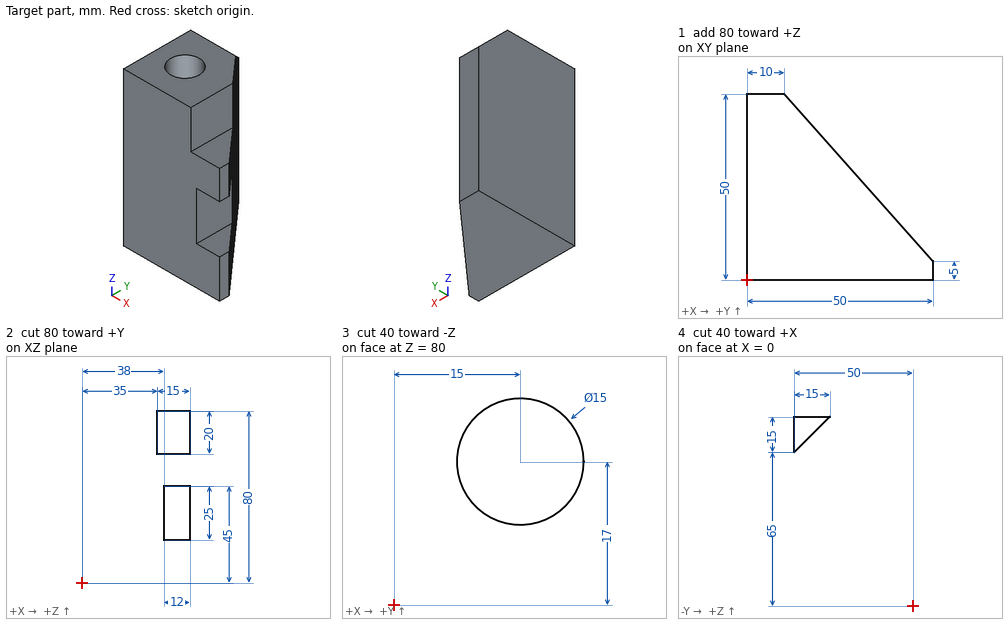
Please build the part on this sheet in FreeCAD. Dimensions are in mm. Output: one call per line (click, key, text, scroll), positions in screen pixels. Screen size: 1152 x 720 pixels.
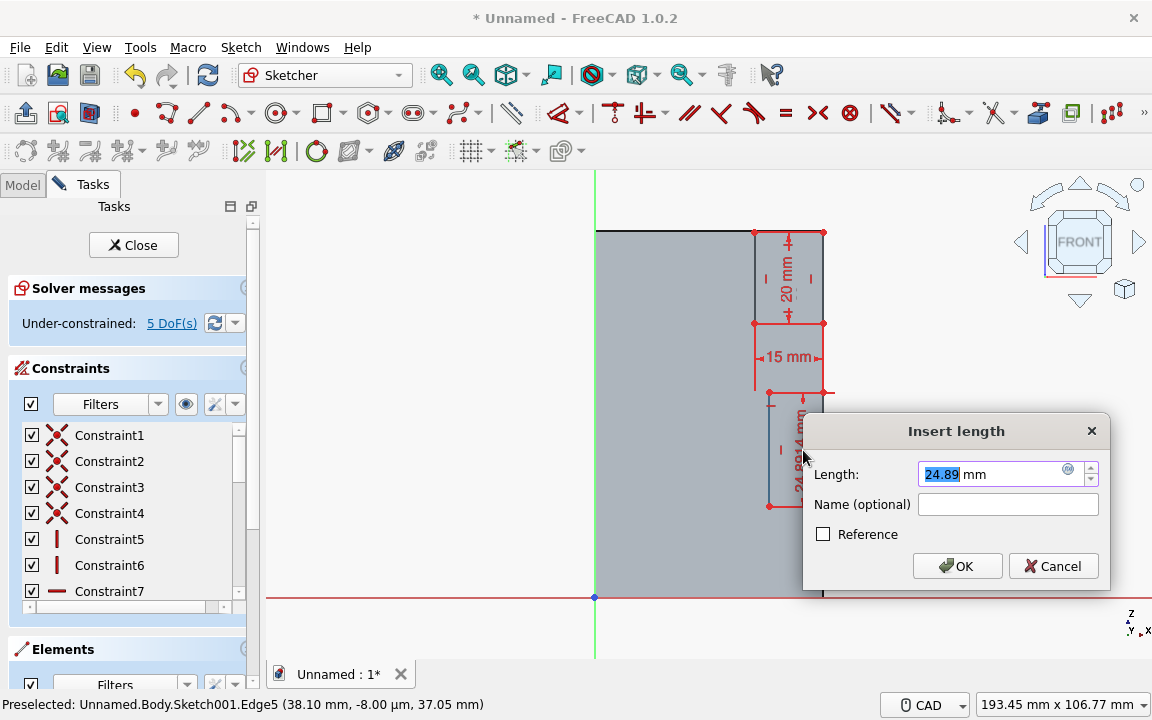
text(25)
key(Return)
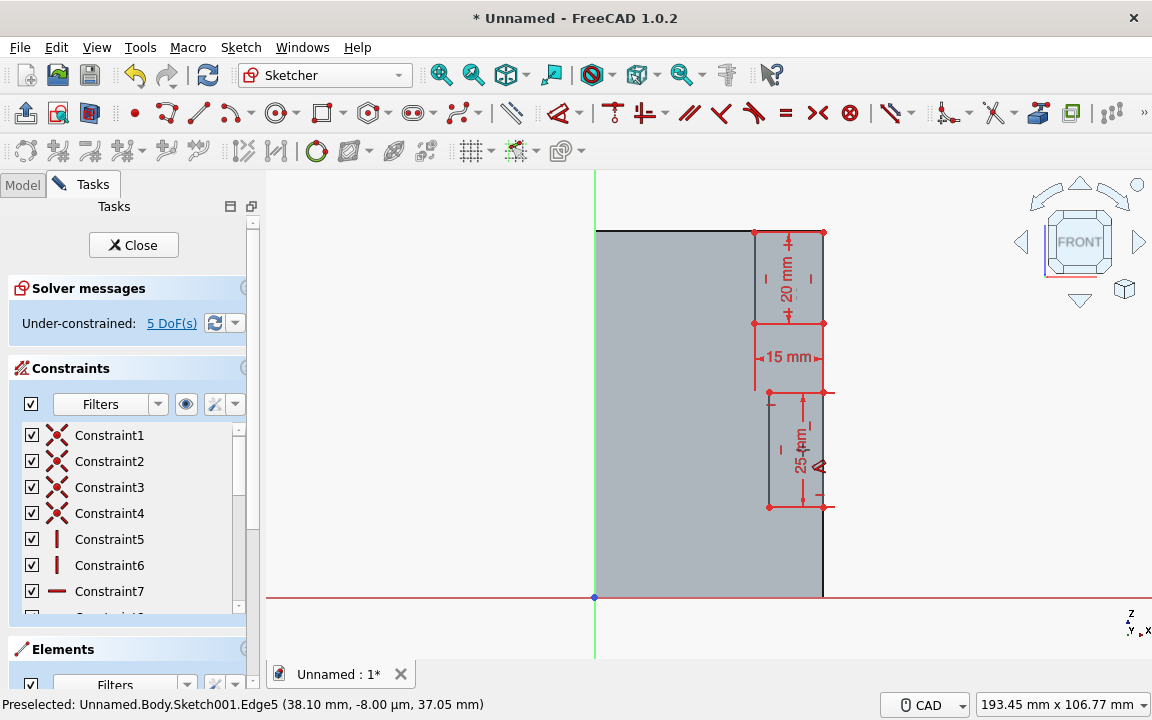
click(785, 507)
click(796, 541)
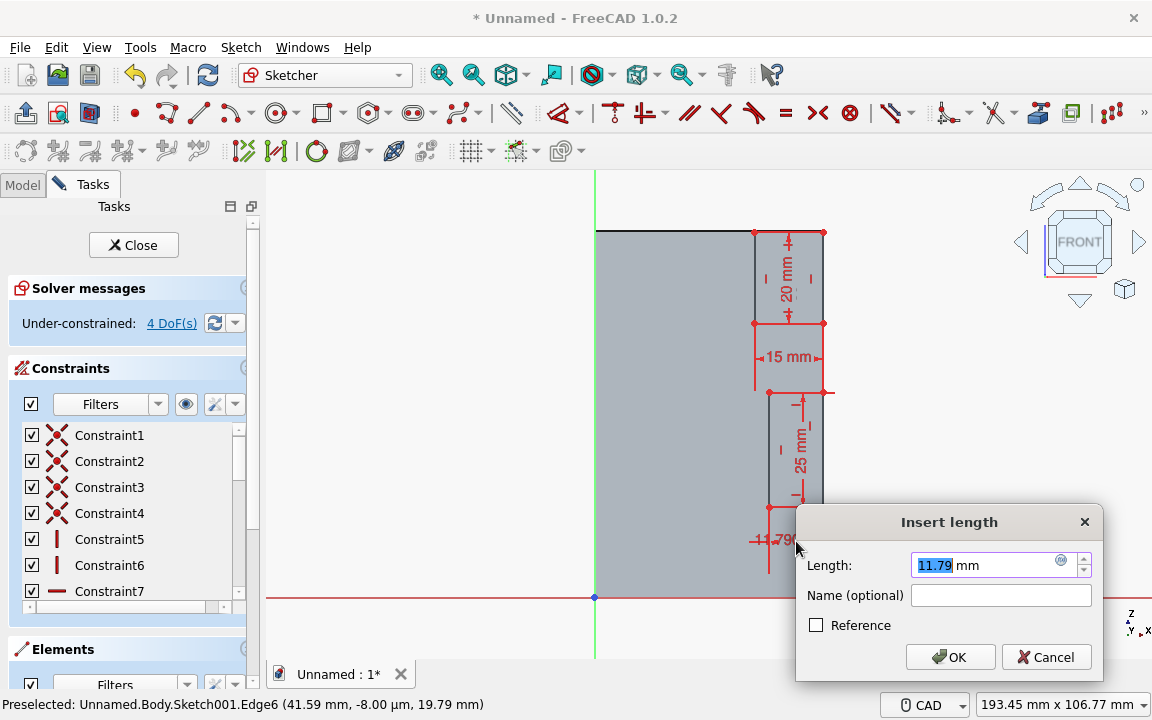
text(12)
key(Return)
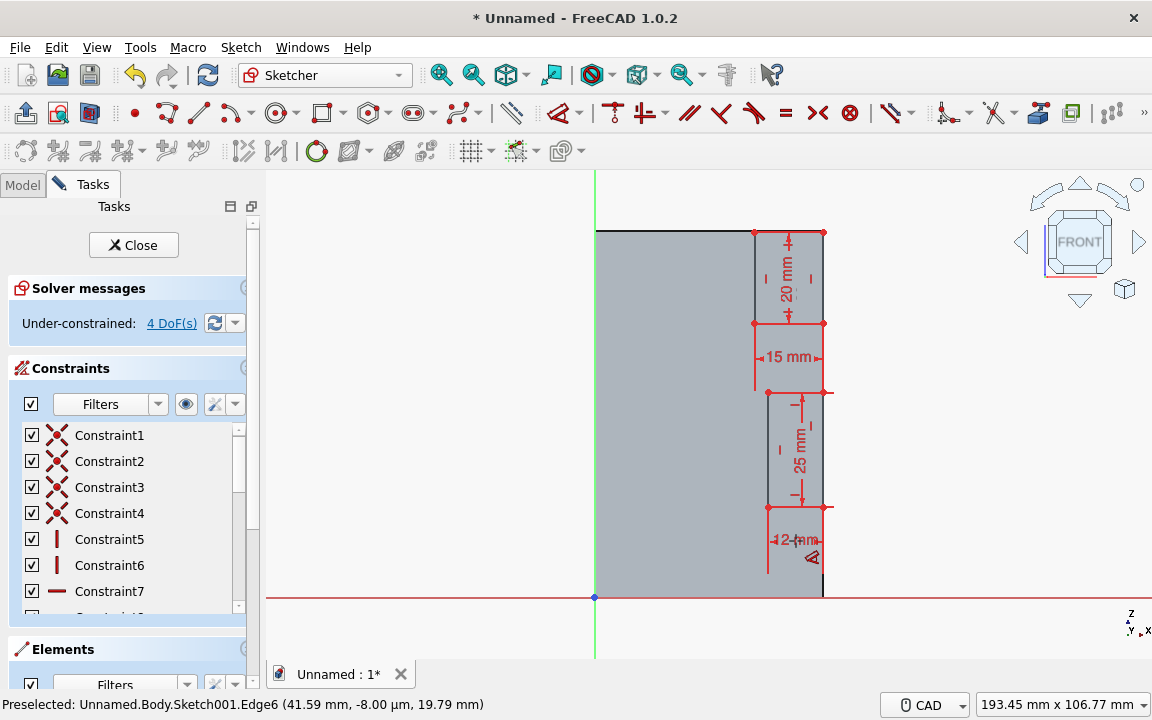
click(755, 232)
click(675, 198)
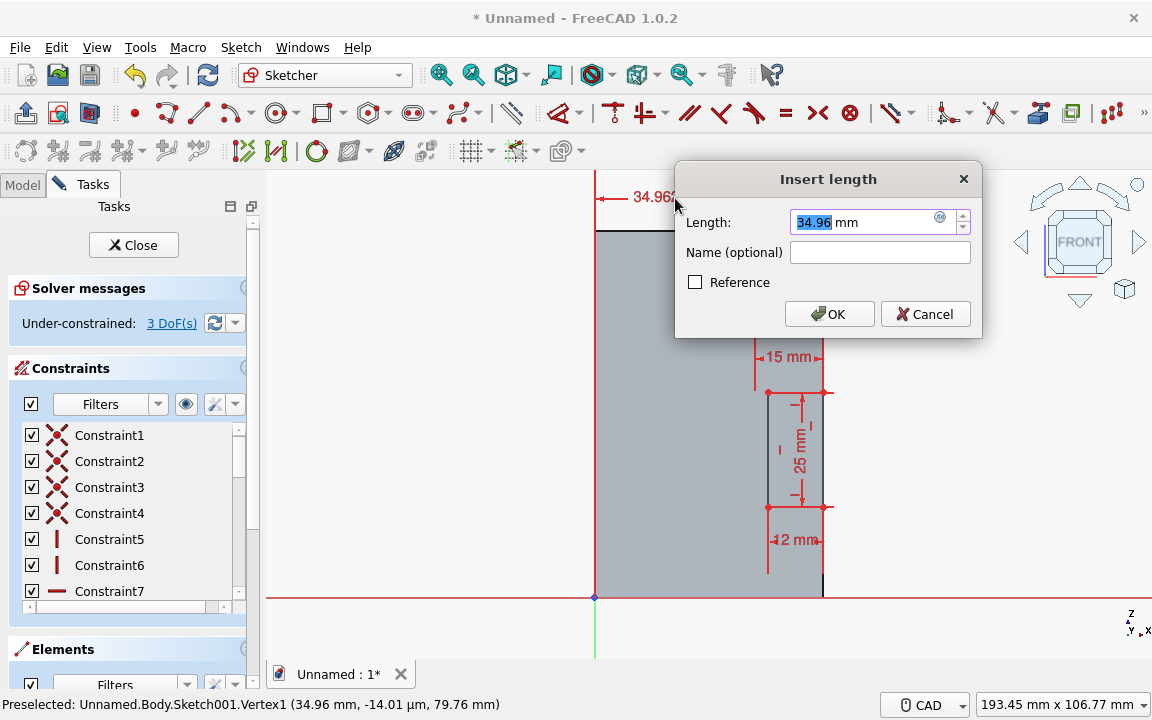
text(35)
key(Return)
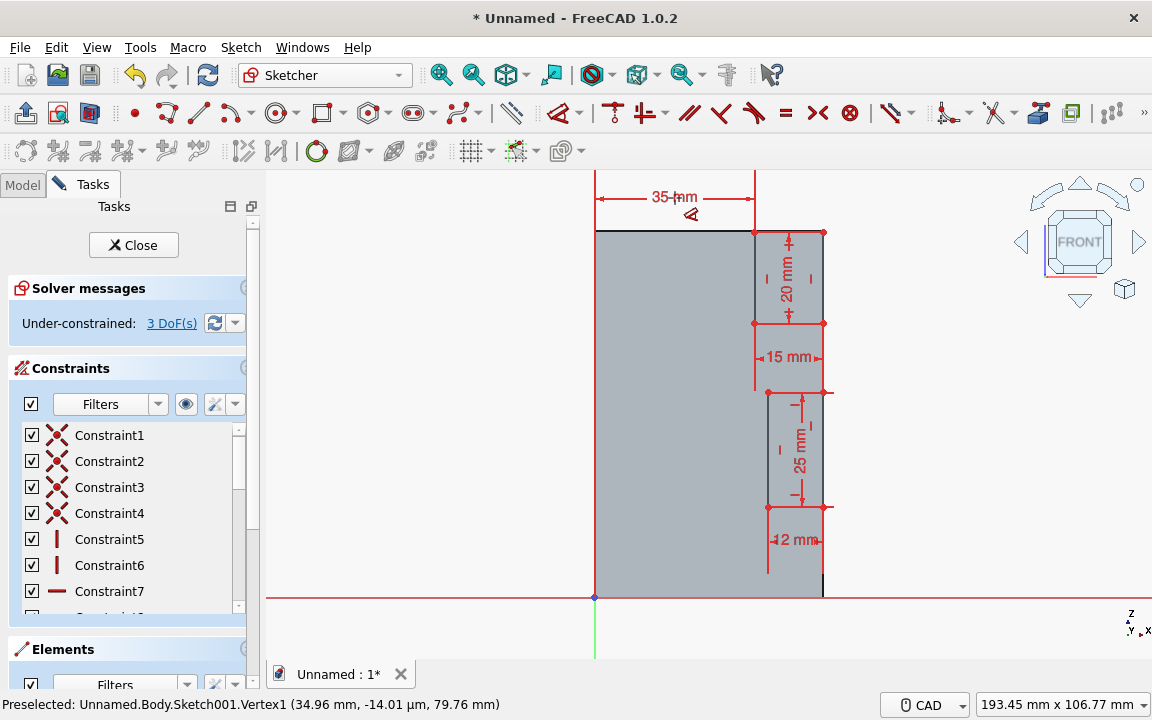
click(755, 232)
click(561, 415)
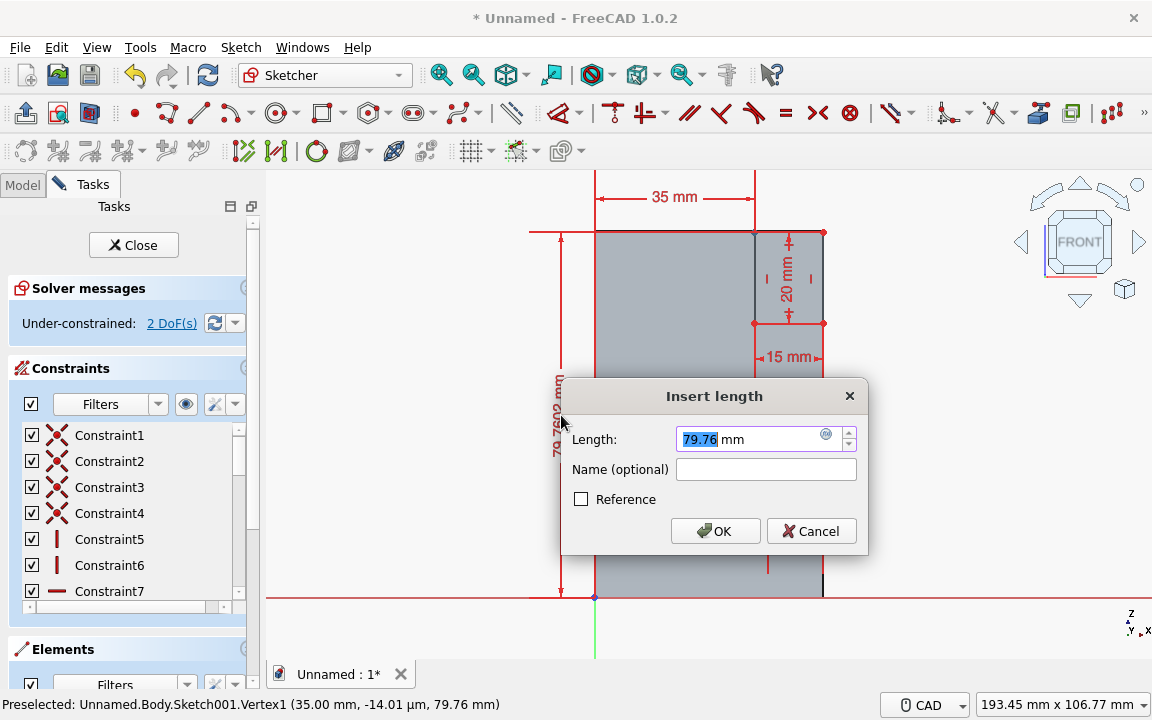
text(80)
key(Return)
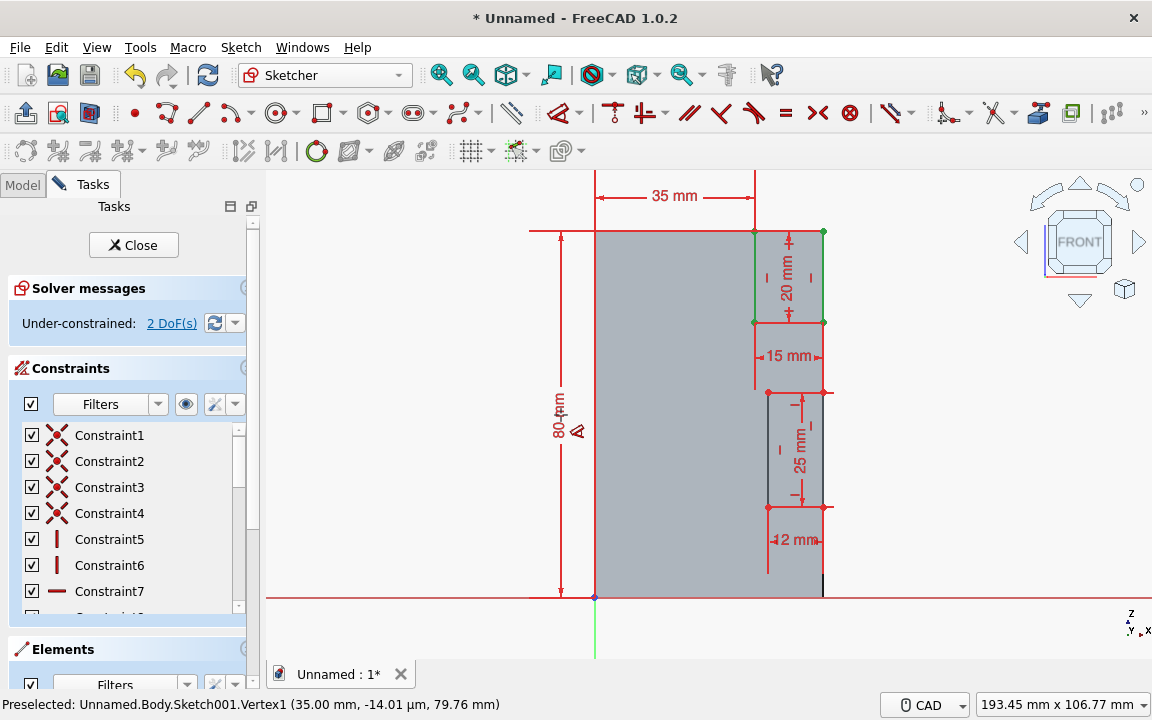
click(768, 393)
click(681, 359)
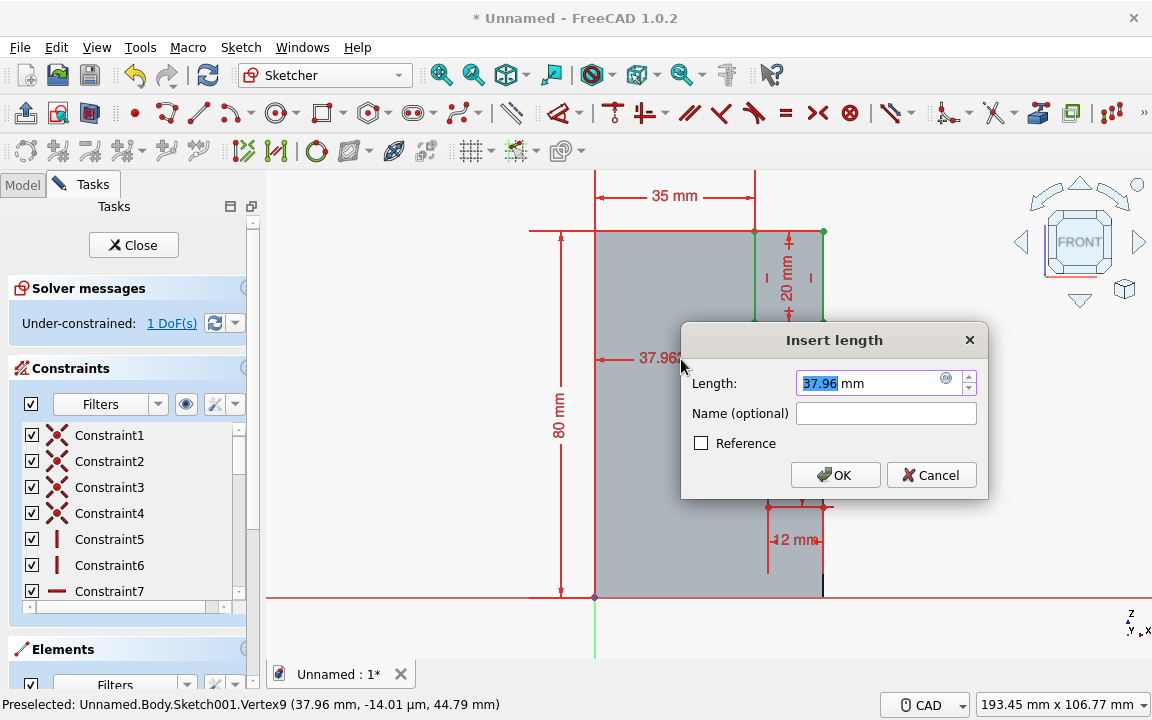
text(38)
key(Return)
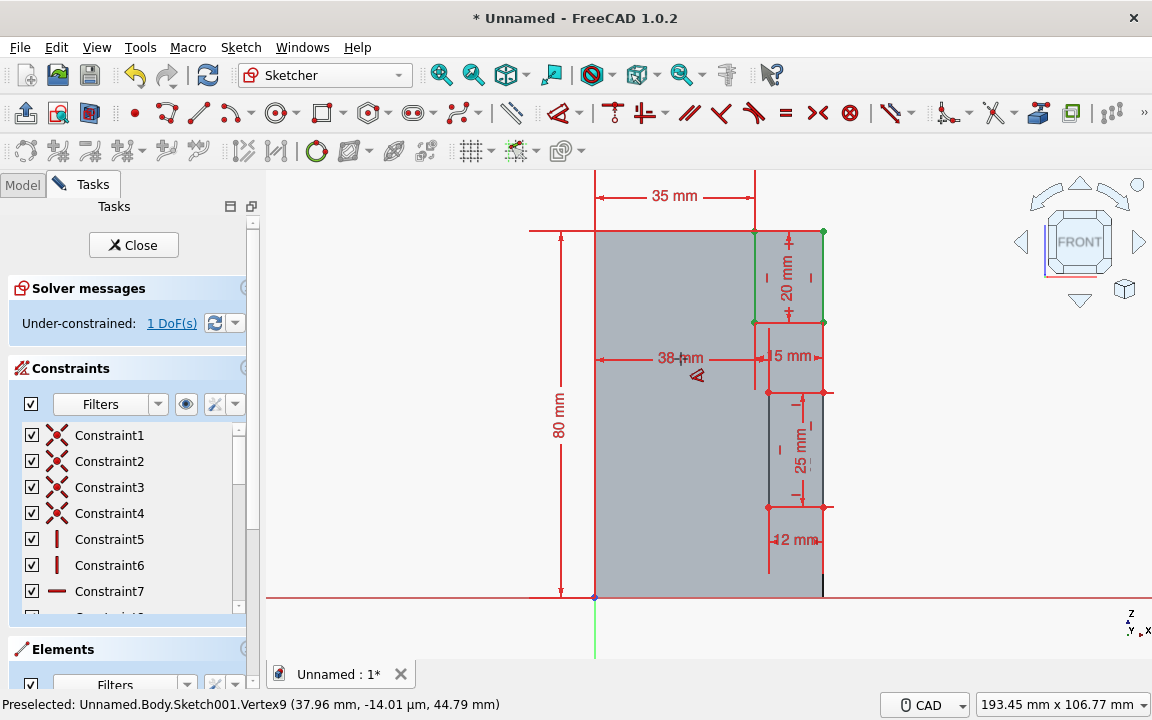
click(769, 393)
click(561, 495)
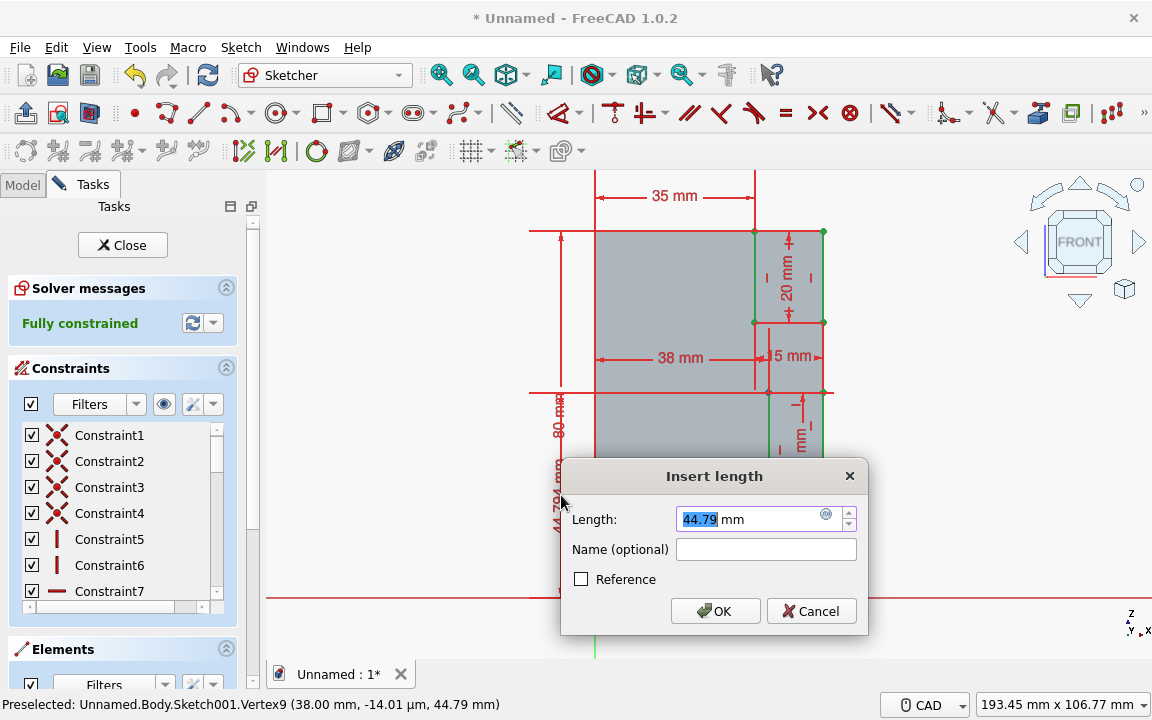
text(45)
key(Return)
key(Escape)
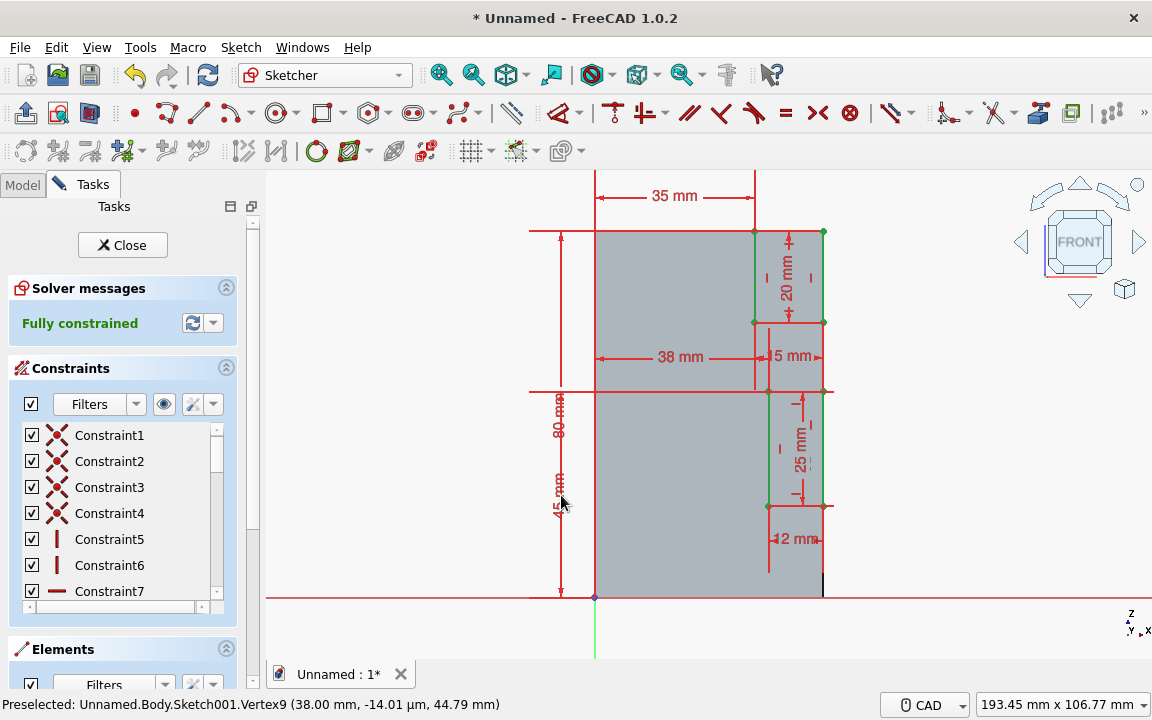
click(123, 245)